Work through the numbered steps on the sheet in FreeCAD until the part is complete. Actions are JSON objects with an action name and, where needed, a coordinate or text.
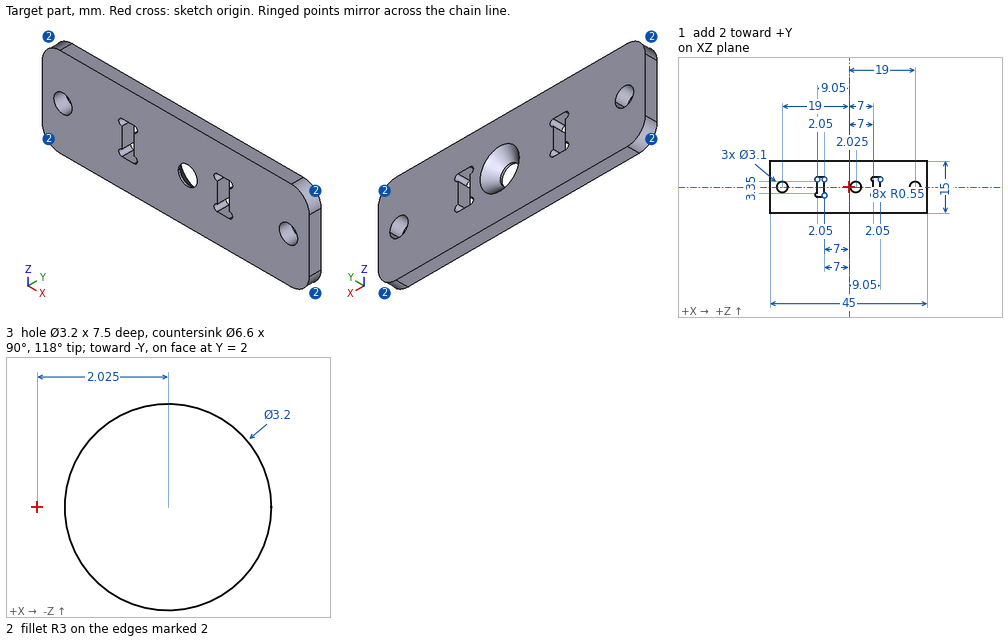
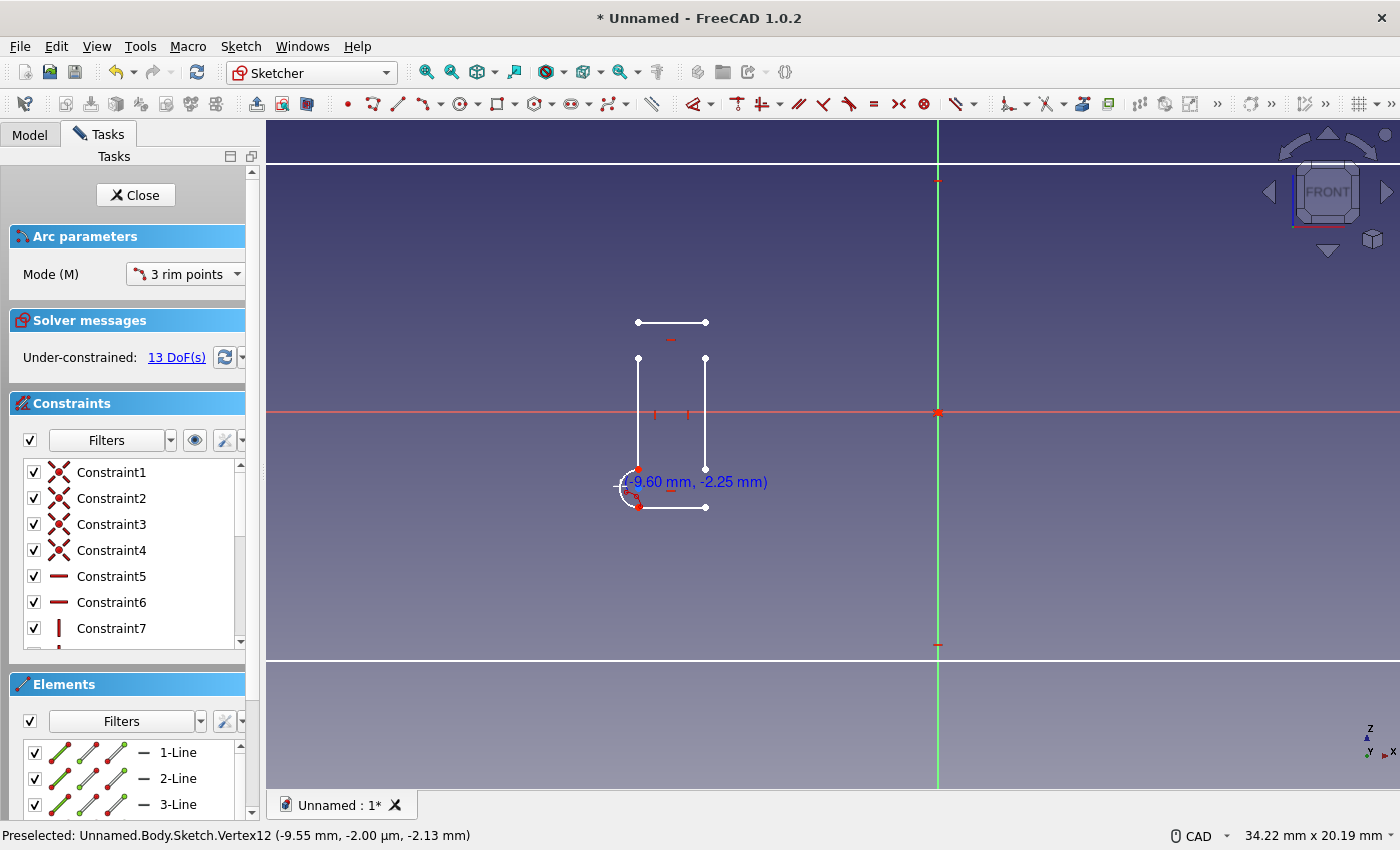
{"action": "left_click", "coordinate": [705, 508]}
{"action": "left_click", "coordinate": [705, 470]}
{"action": "left_click", "coordinate": [724, 486]}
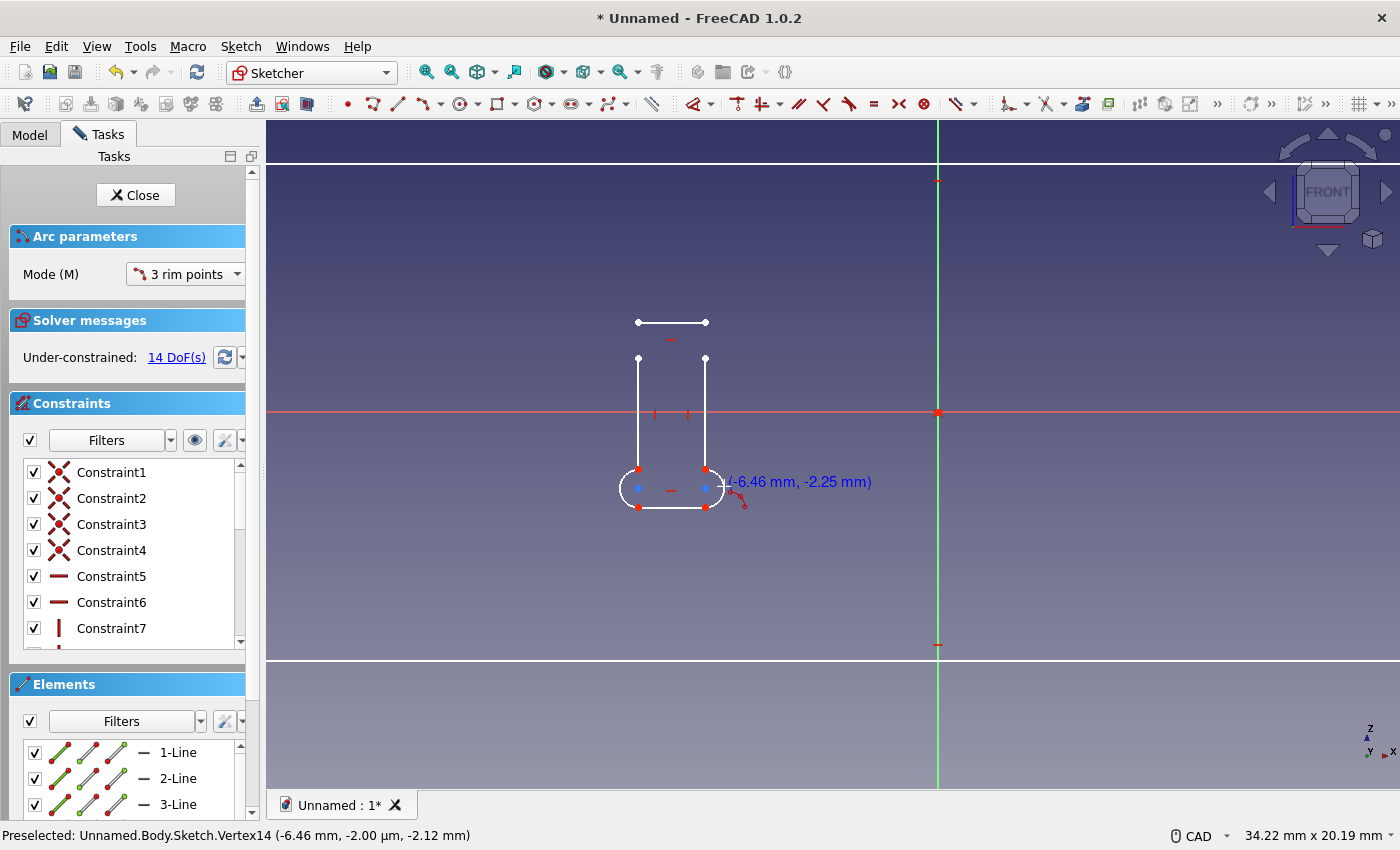
{"action": "left_click", "coordinate": [705, 358]}
{"action": "left_click", "coordinate": [705, 323]}
{"action": "left_click", "coordinate": [724, 339]}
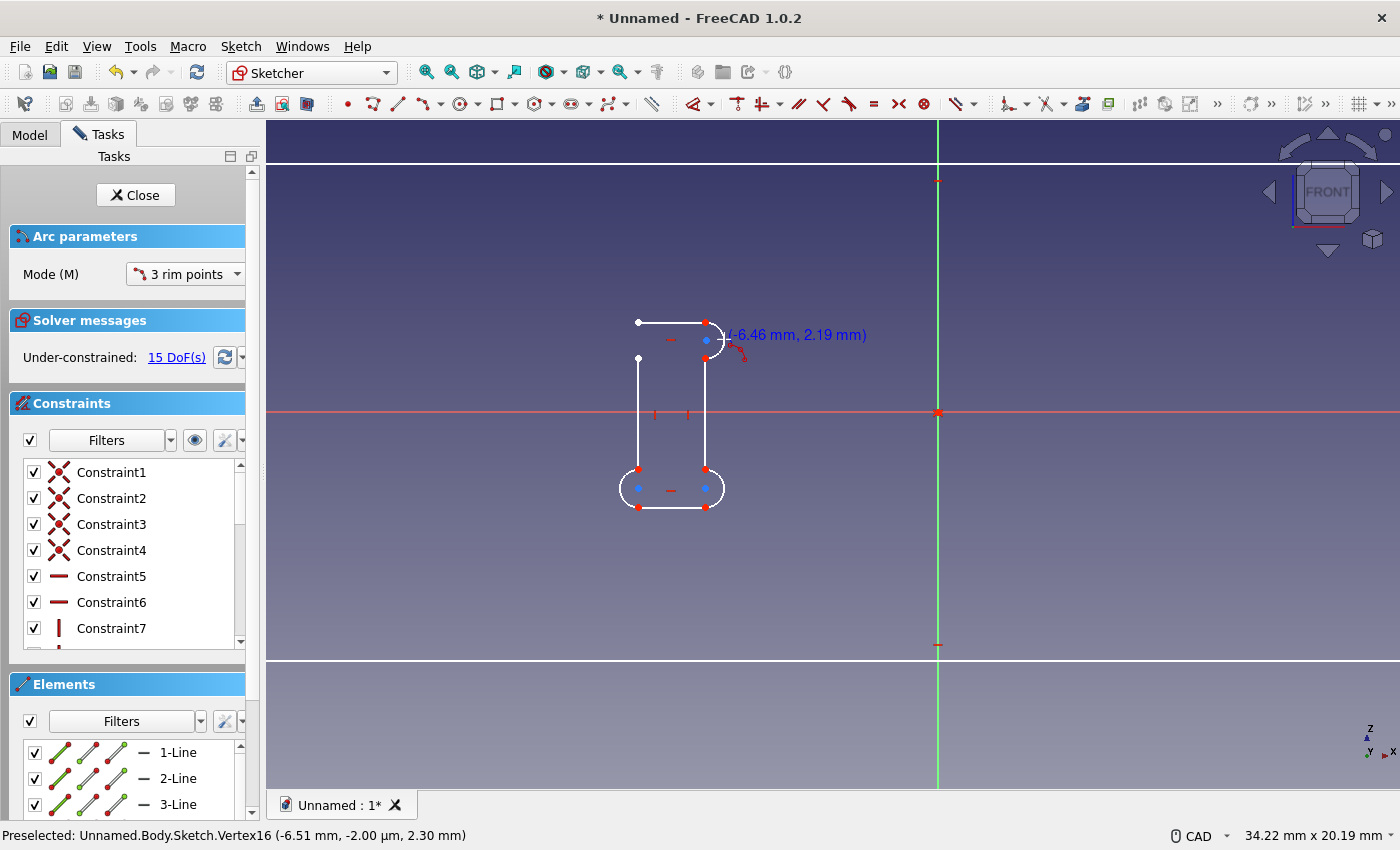
{"action": "left_click", "coordinate": [638, 323]}
{"action": "left_click", "coordinate": [638, 358]}
{"action": "left_click", "coordinate": [620, 339]}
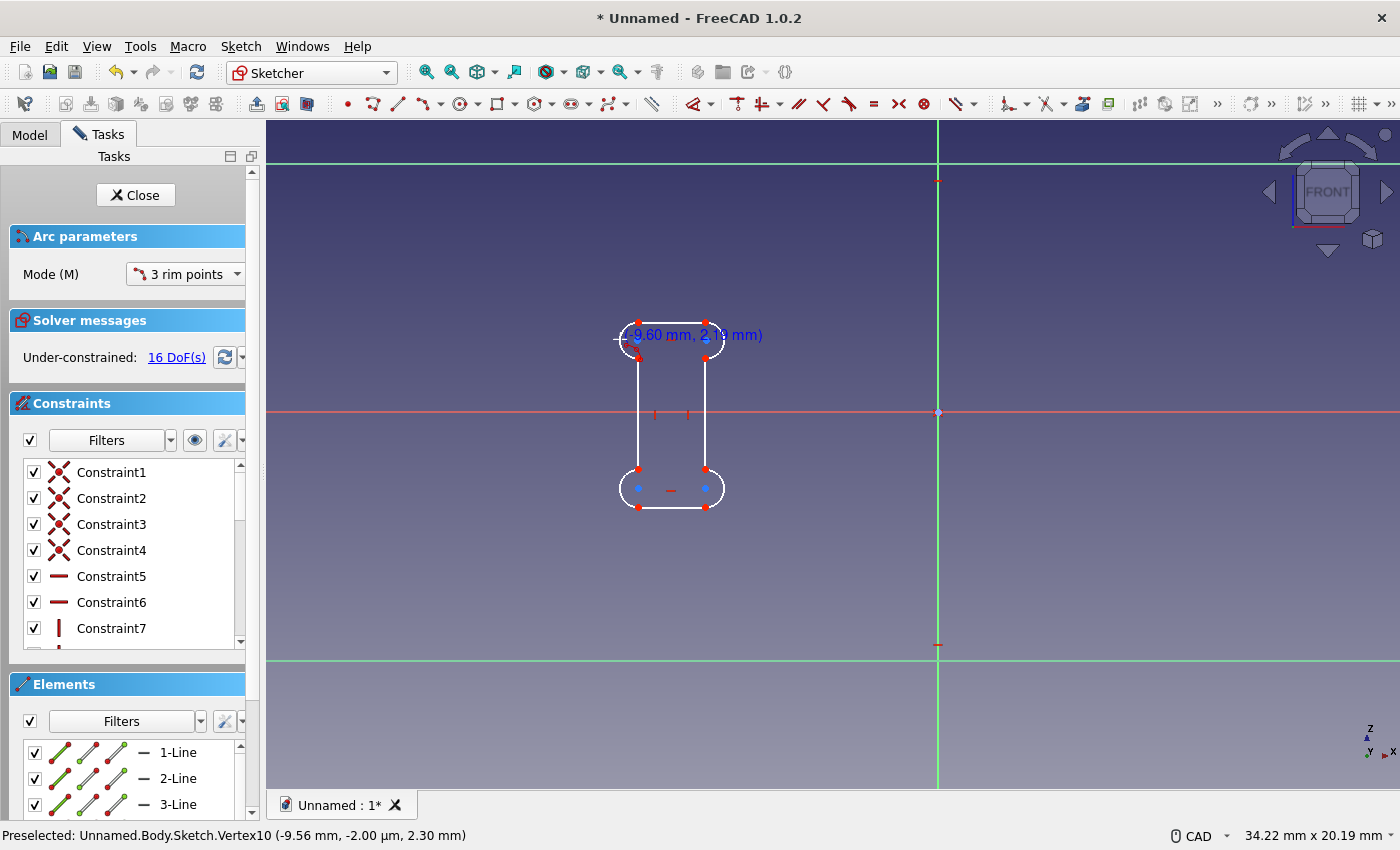
{"action": "left_click", "coordinate": [398, 104]}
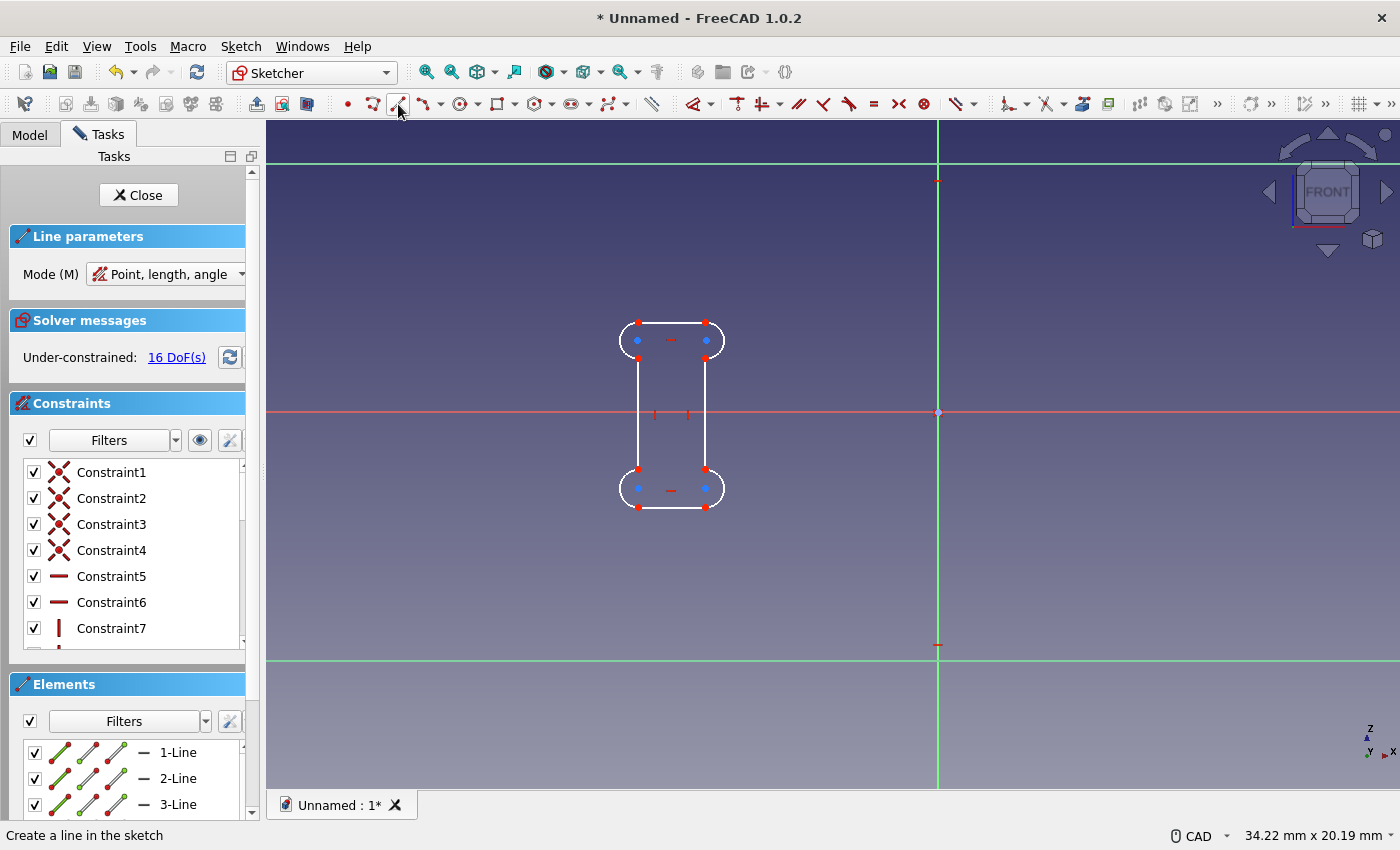
{"action": "left_click", "coordinate": [1170, 357]}
{"action": "left_click", "coordinate": [1170, 468]}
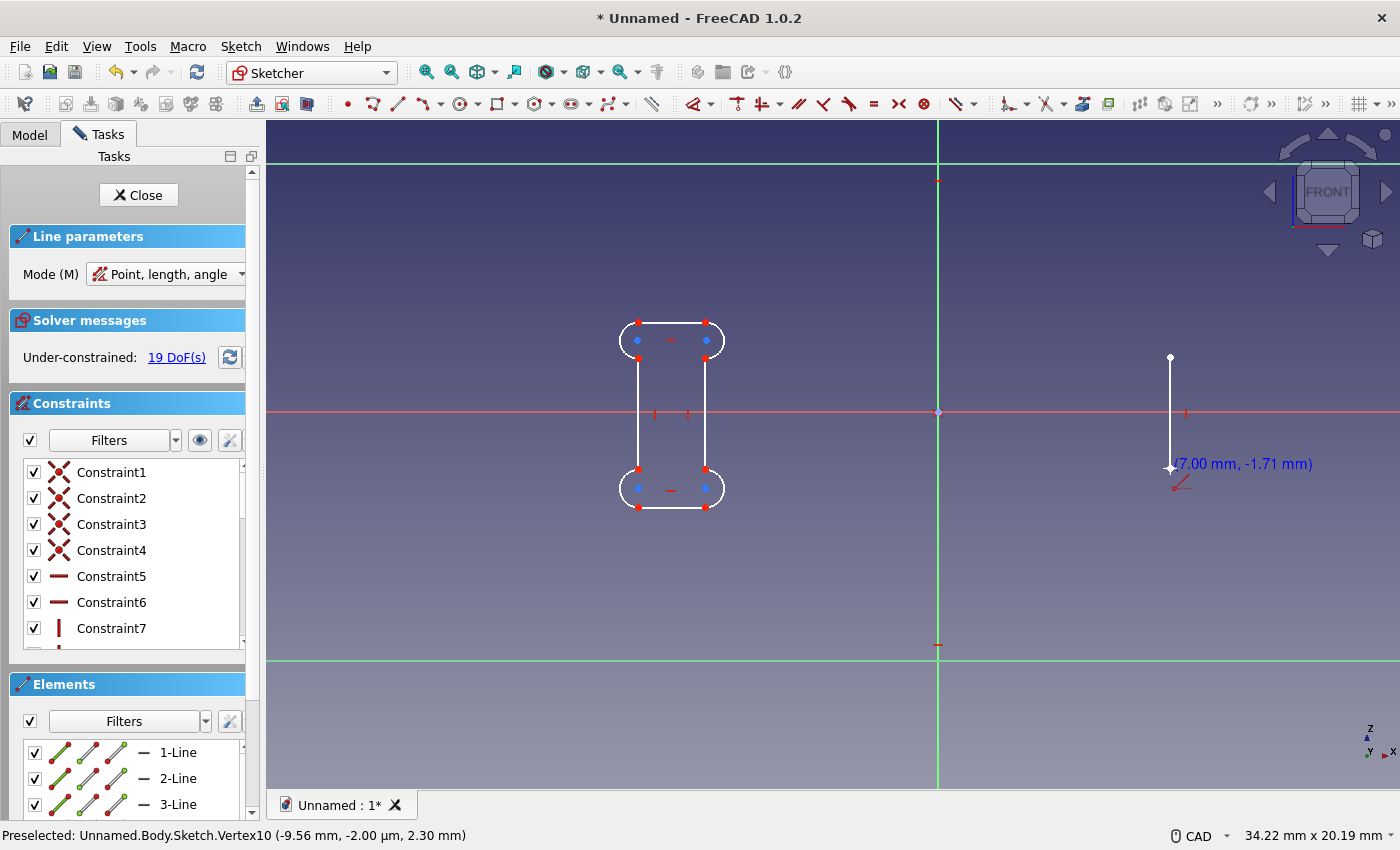
{"action": "left_click", "coordinate": [1170, 504]}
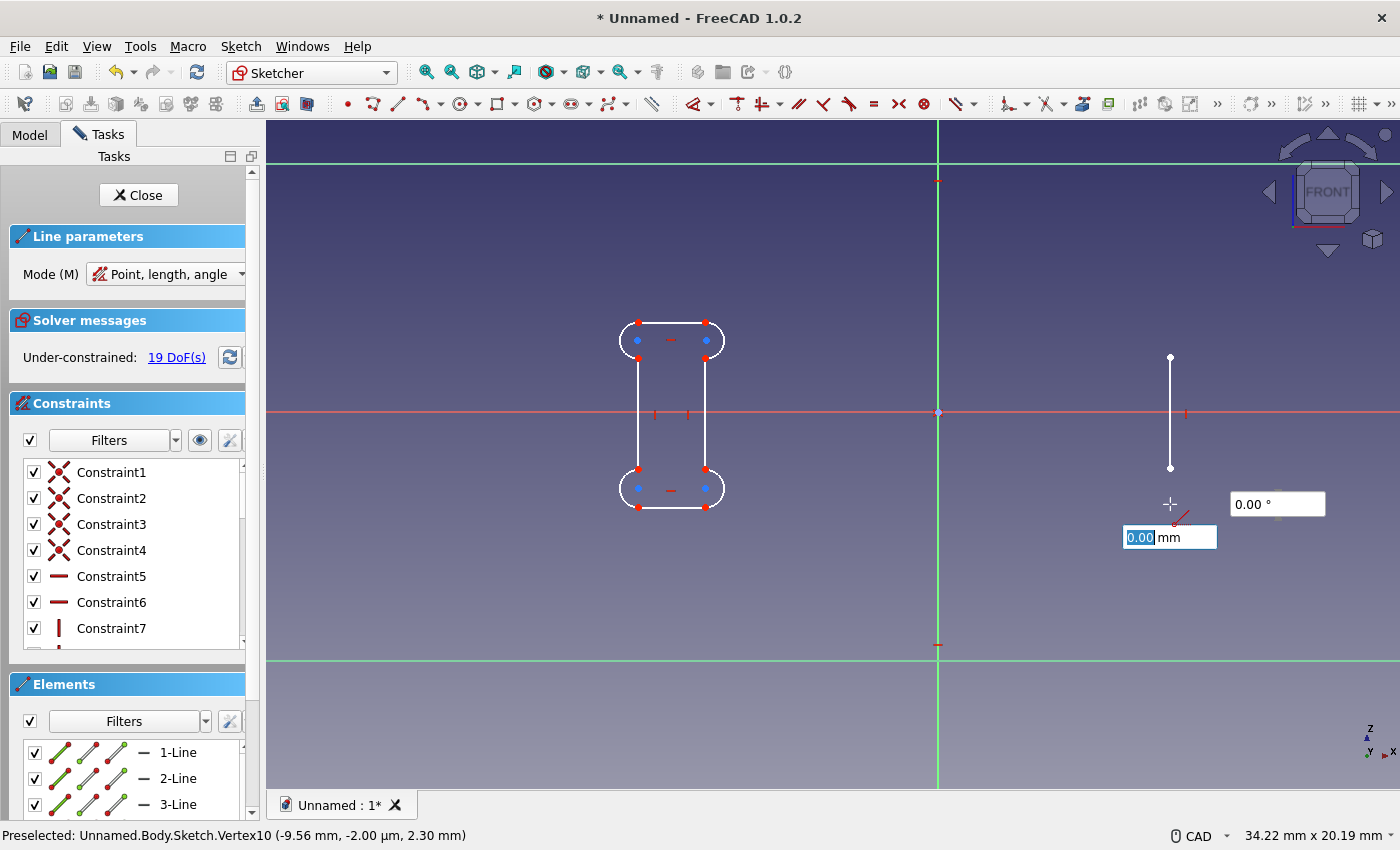
{"action": "scroll", "coordinate": [623, 489], "scroll_direction": "down", "scroll_amount": 4}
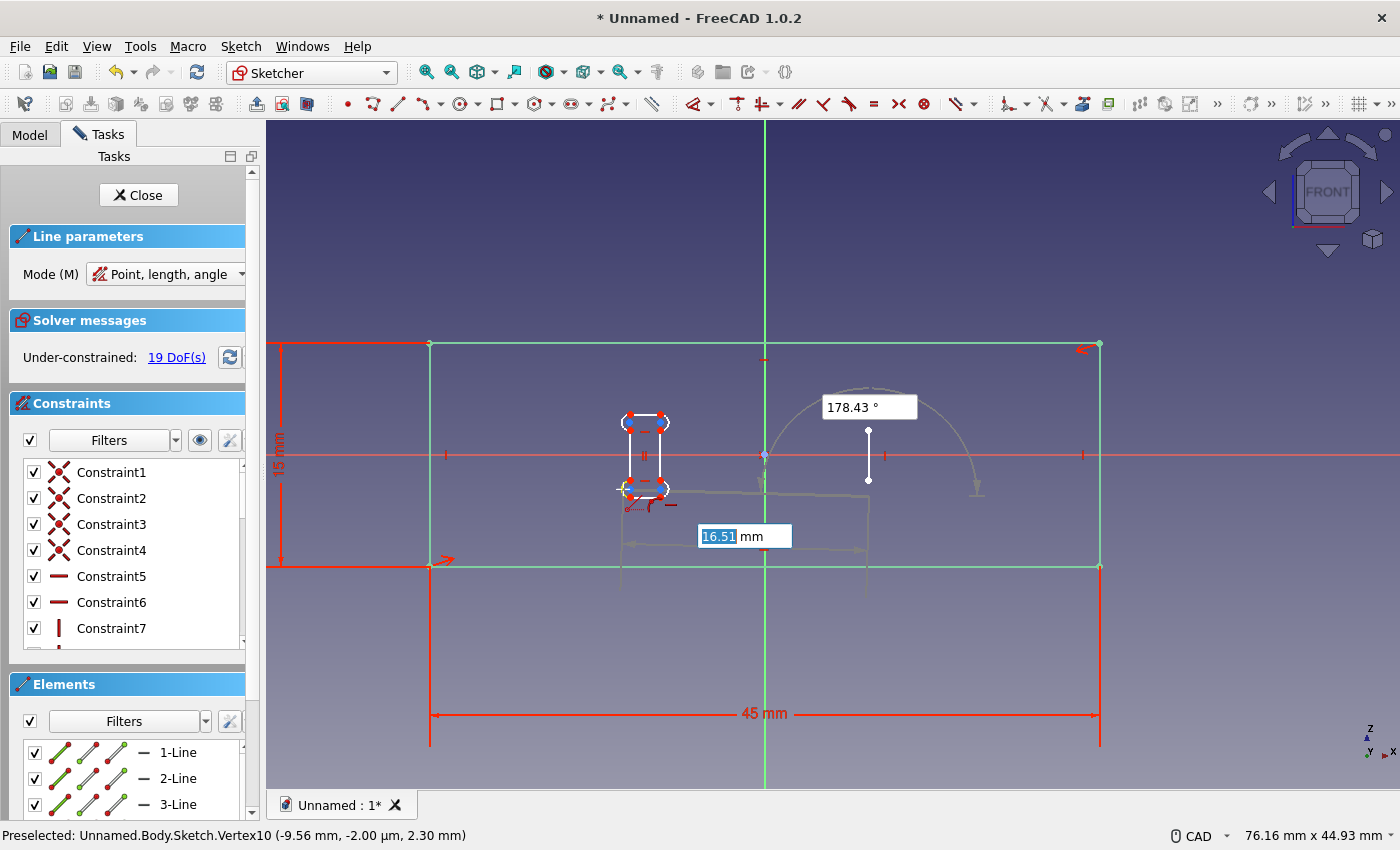
{"action": "left_click", "coordinate": [900, 496]}